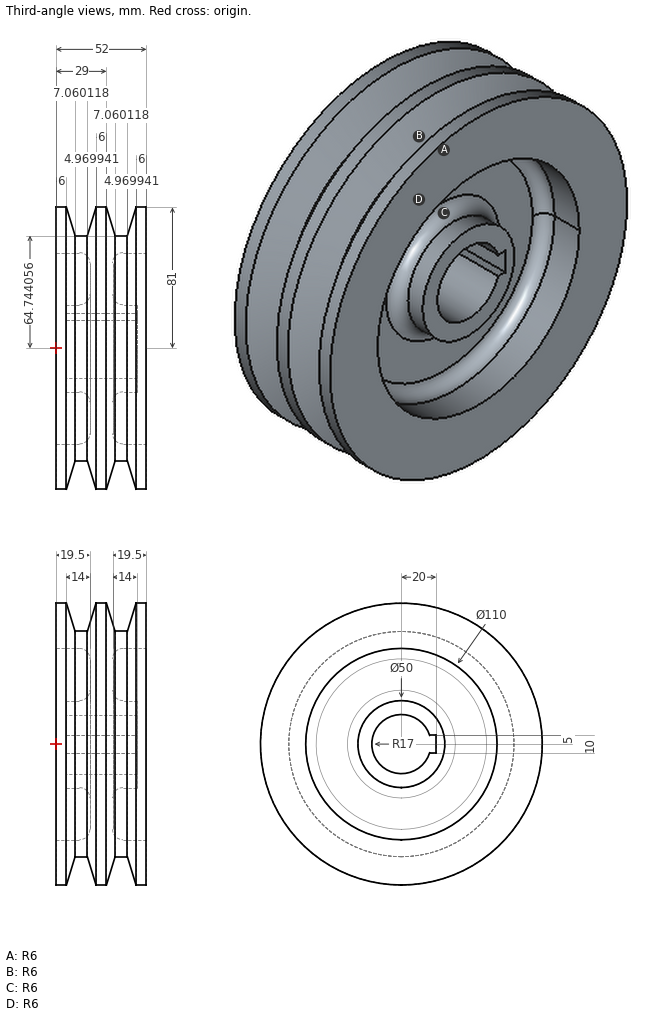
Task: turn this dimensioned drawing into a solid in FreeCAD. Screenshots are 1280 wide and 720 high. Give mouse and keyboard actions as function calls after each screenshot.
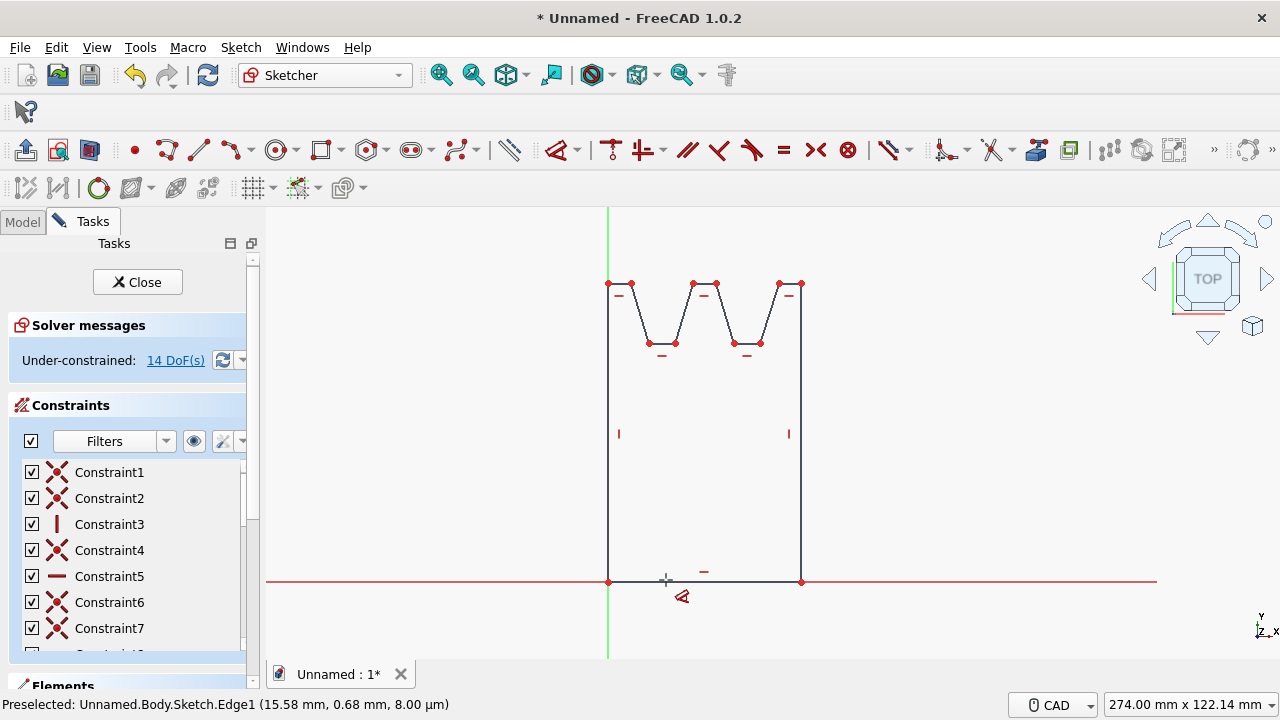
scroll(790, 284, up, 3)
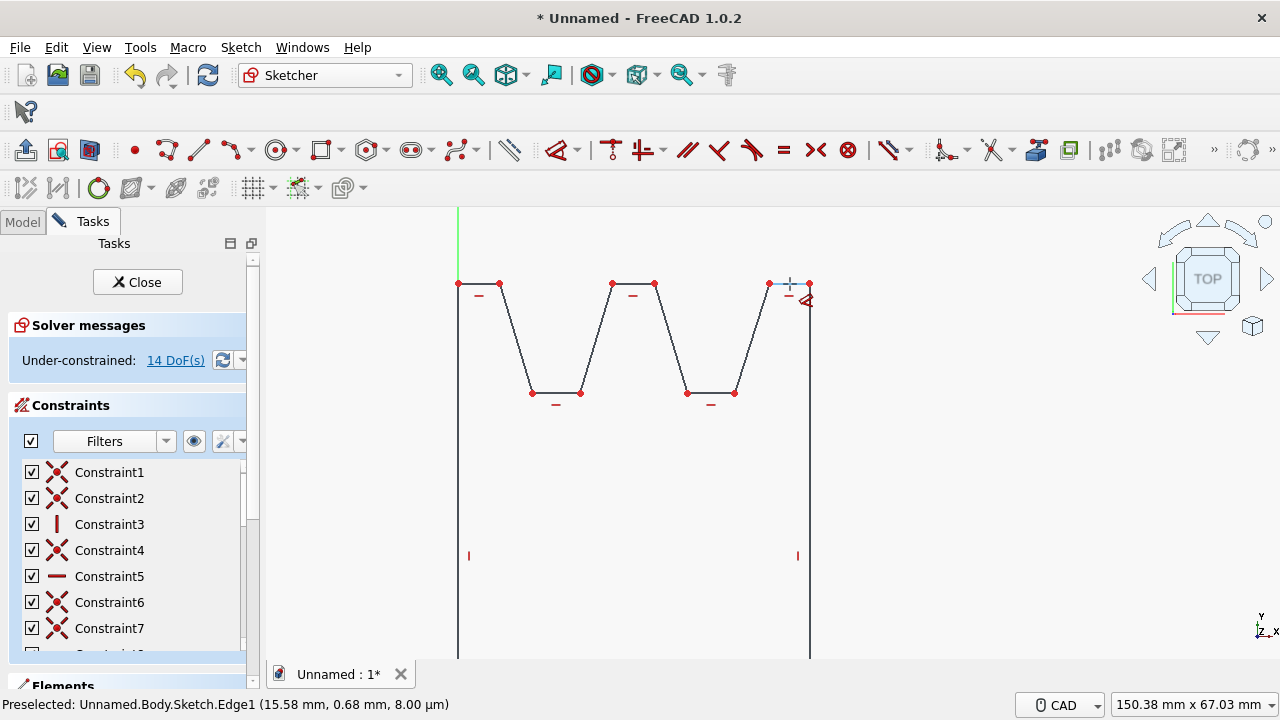
click(790, 284)
click(790, 250)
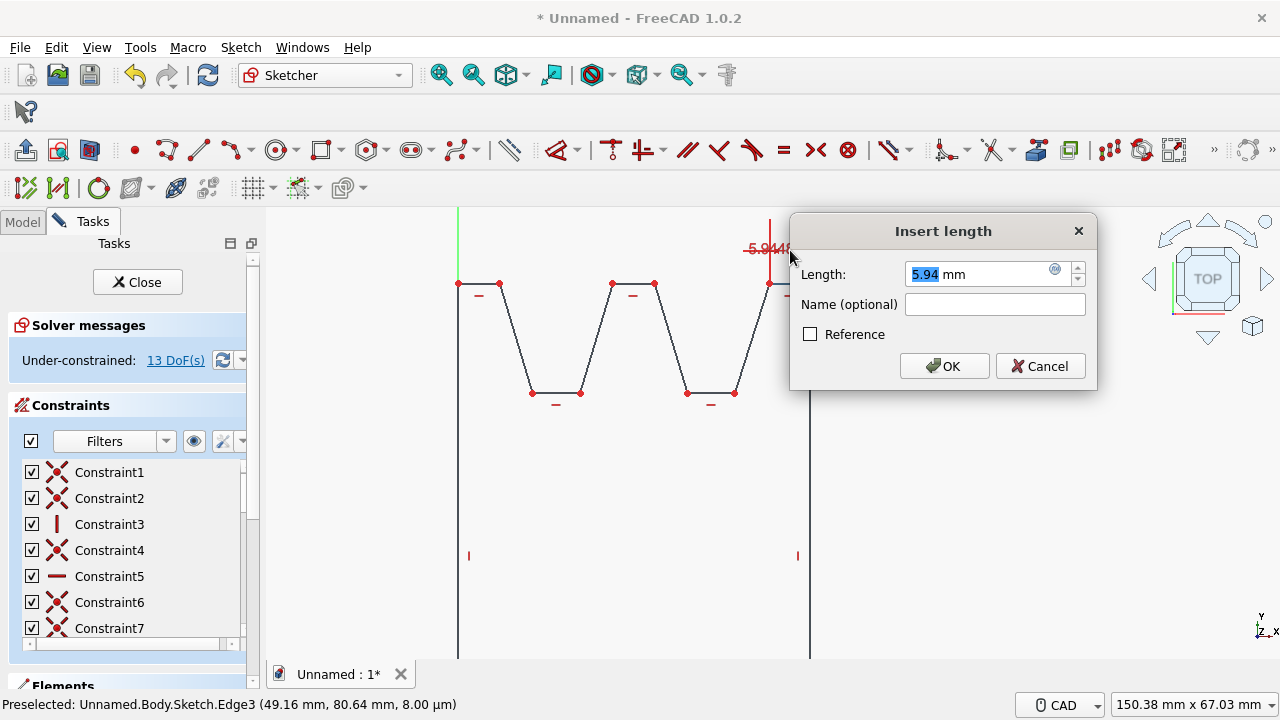
text(6)
key(Return)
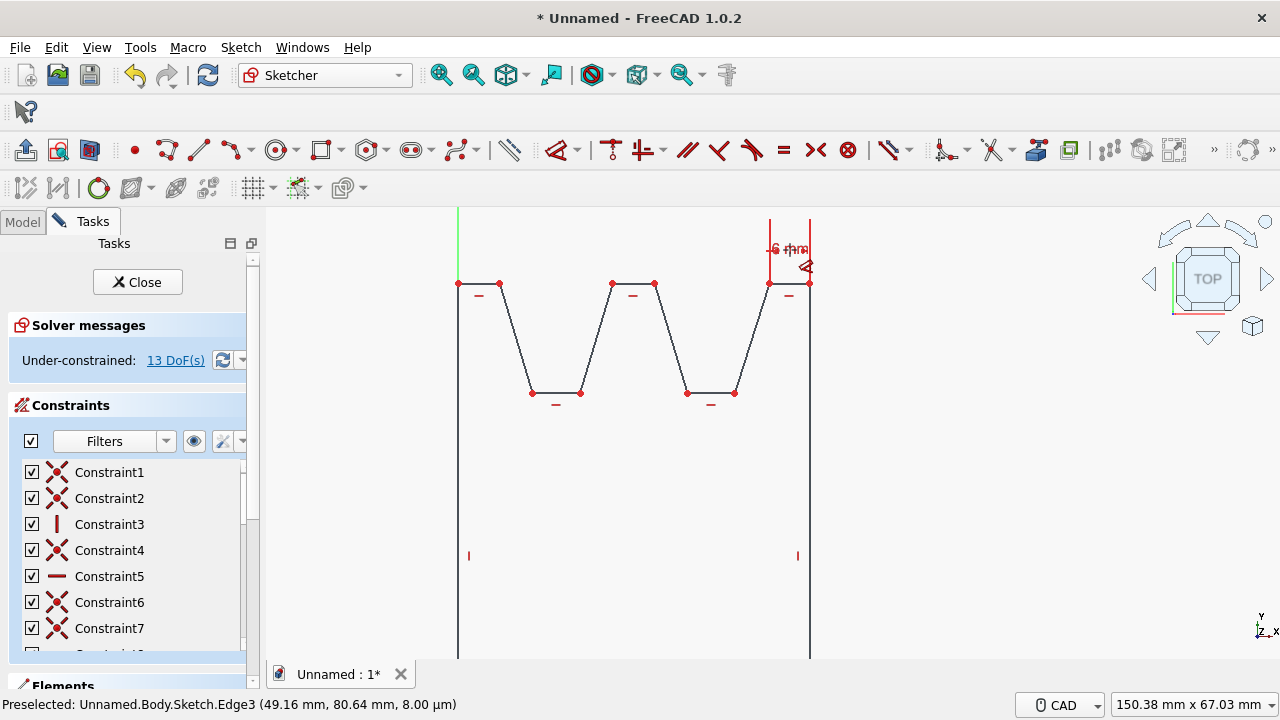
click(642, 284)
click(634, 250)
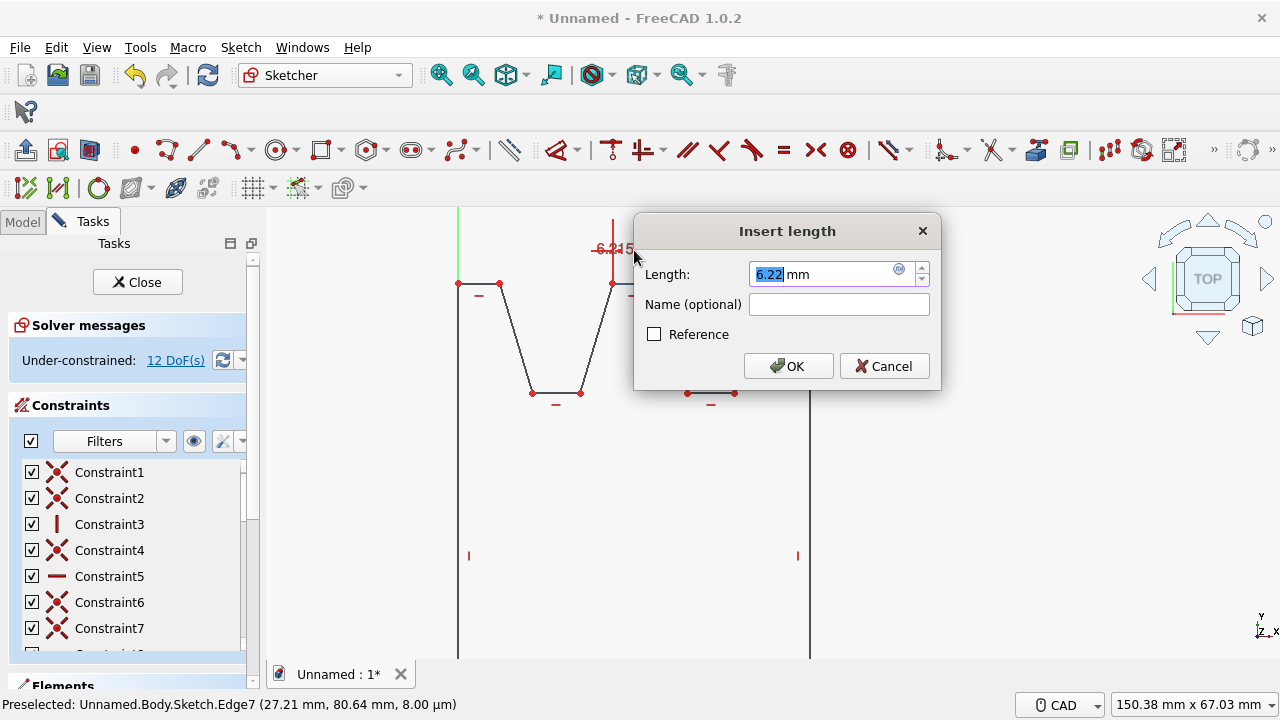
text(6)
key(Return)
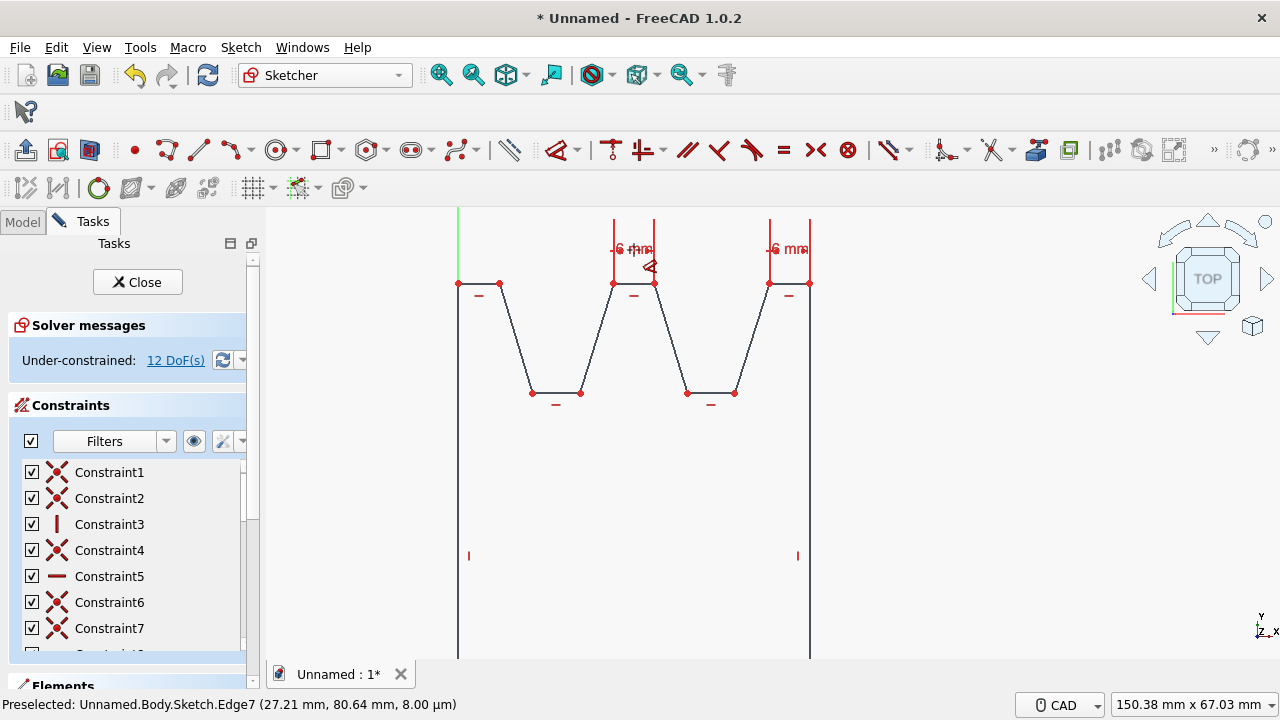
click(487, 284)
click(479, 250)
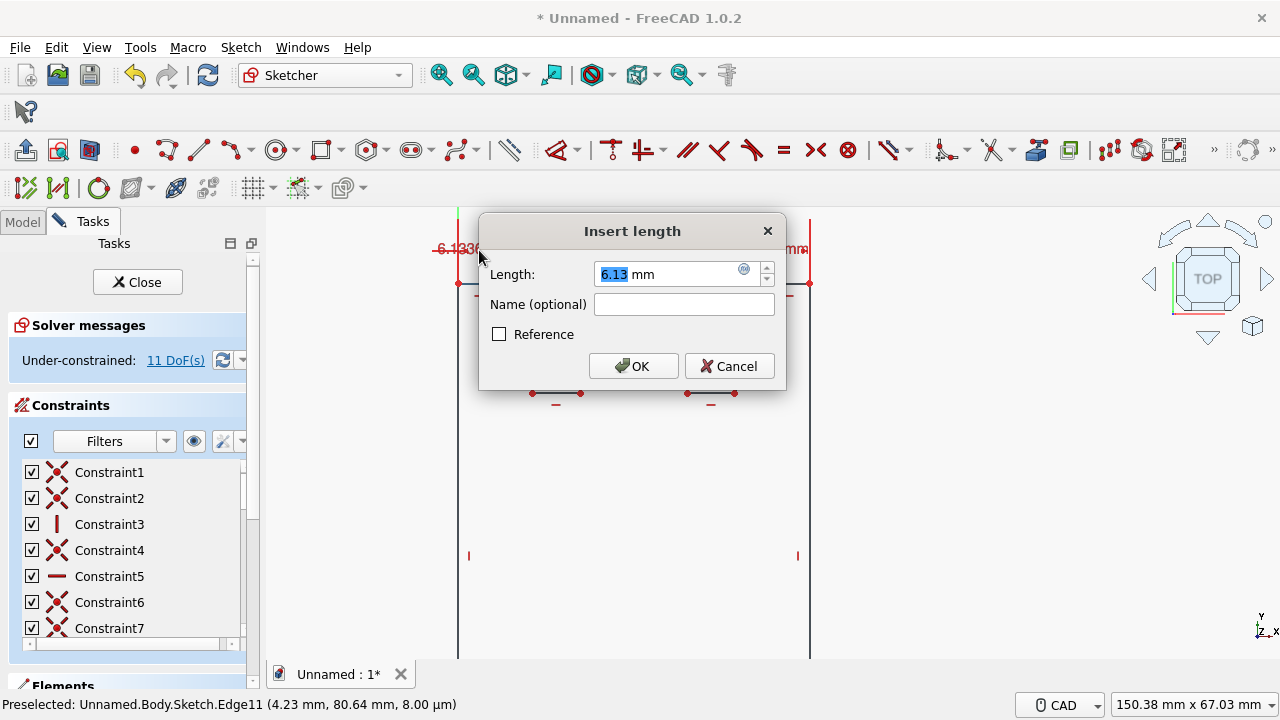
text(6)
key(Return)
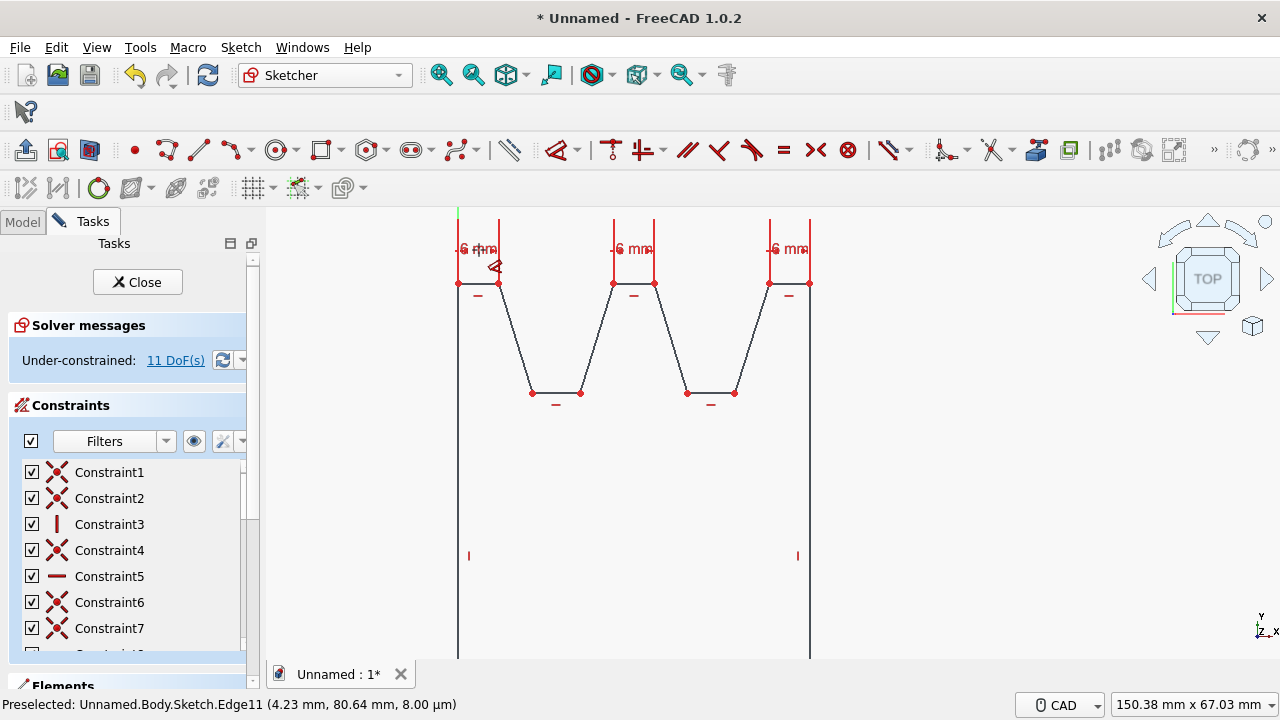
scroll(790, 285, down, 3)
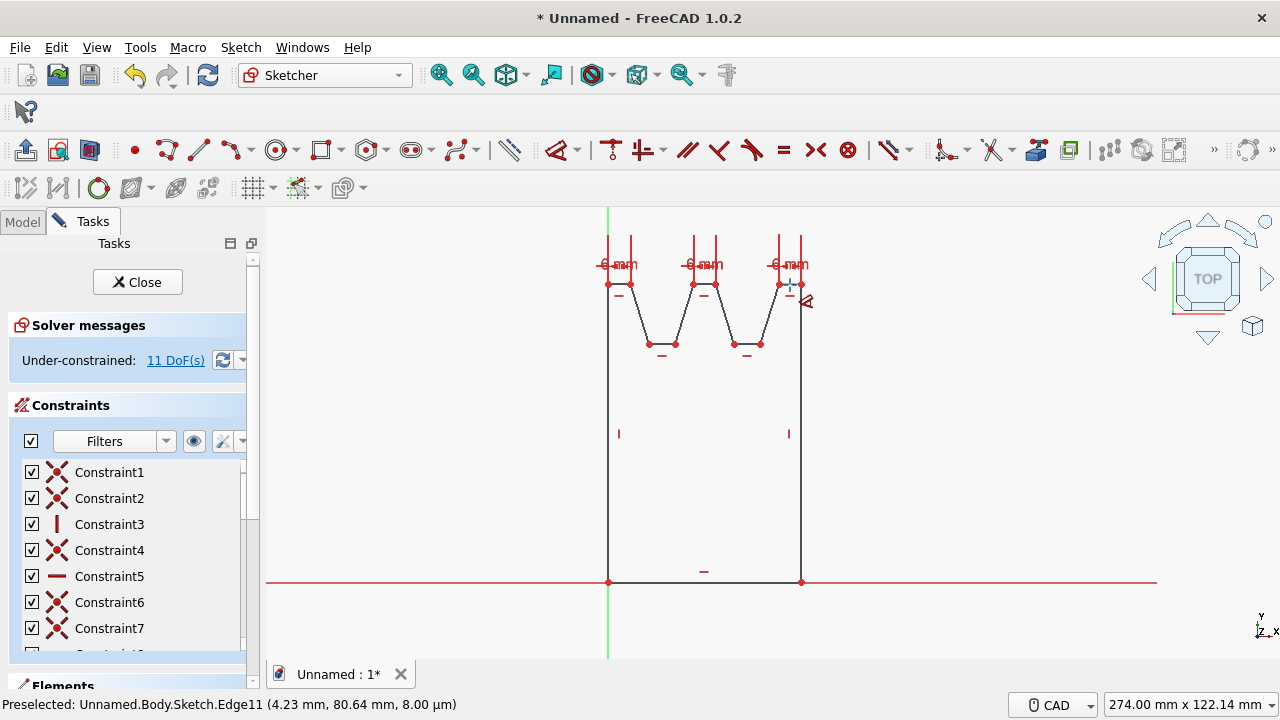
click(666, 583)
click(705, 617)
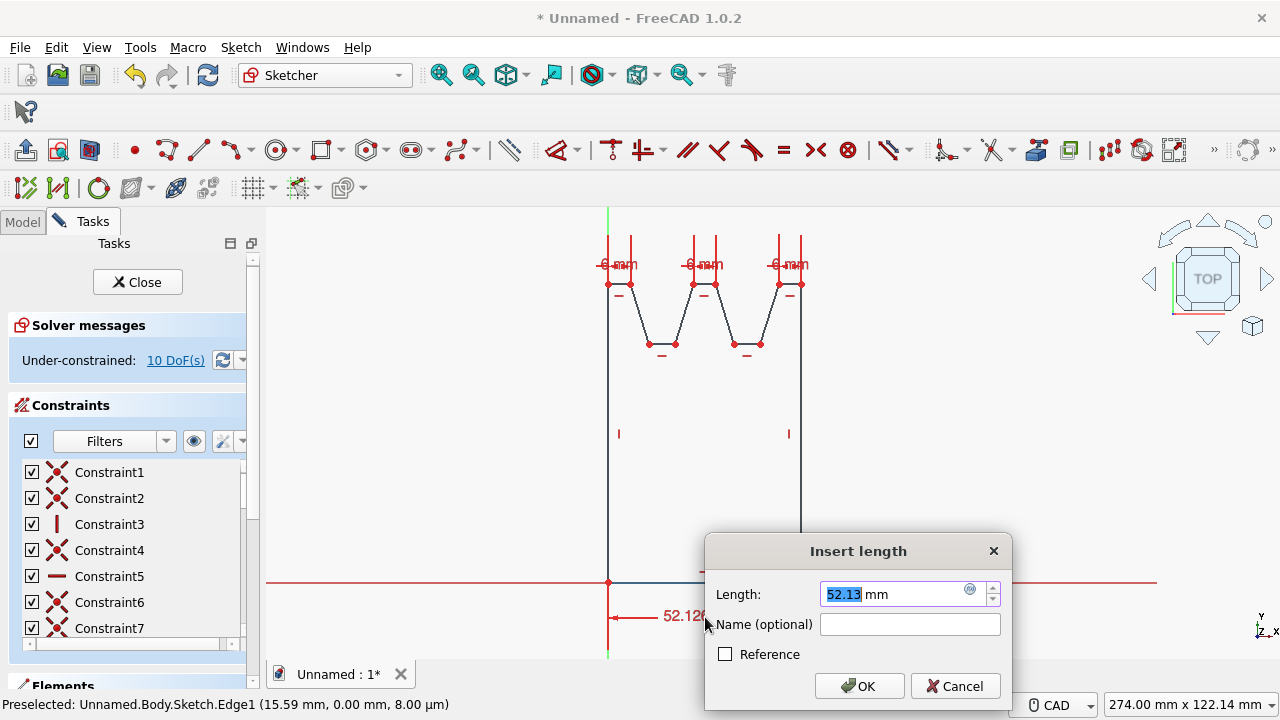
text(52)
key(Return)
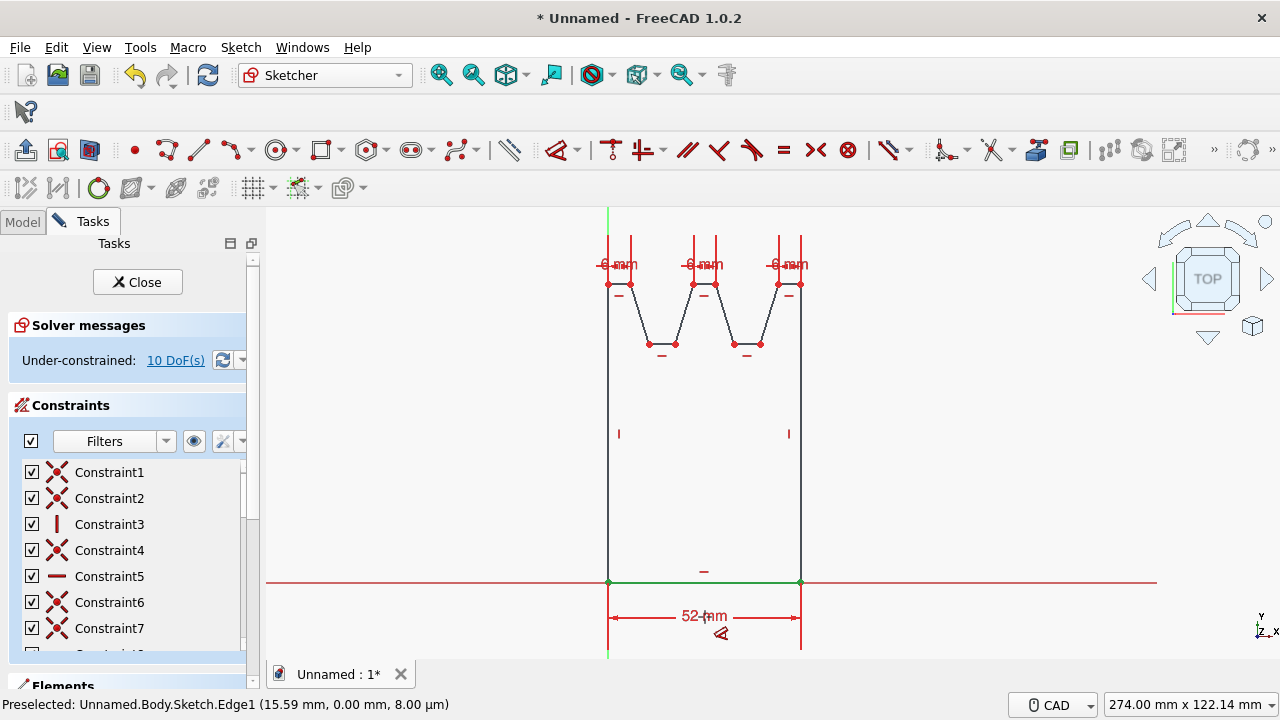
click(801, 493)
click(835, 434)